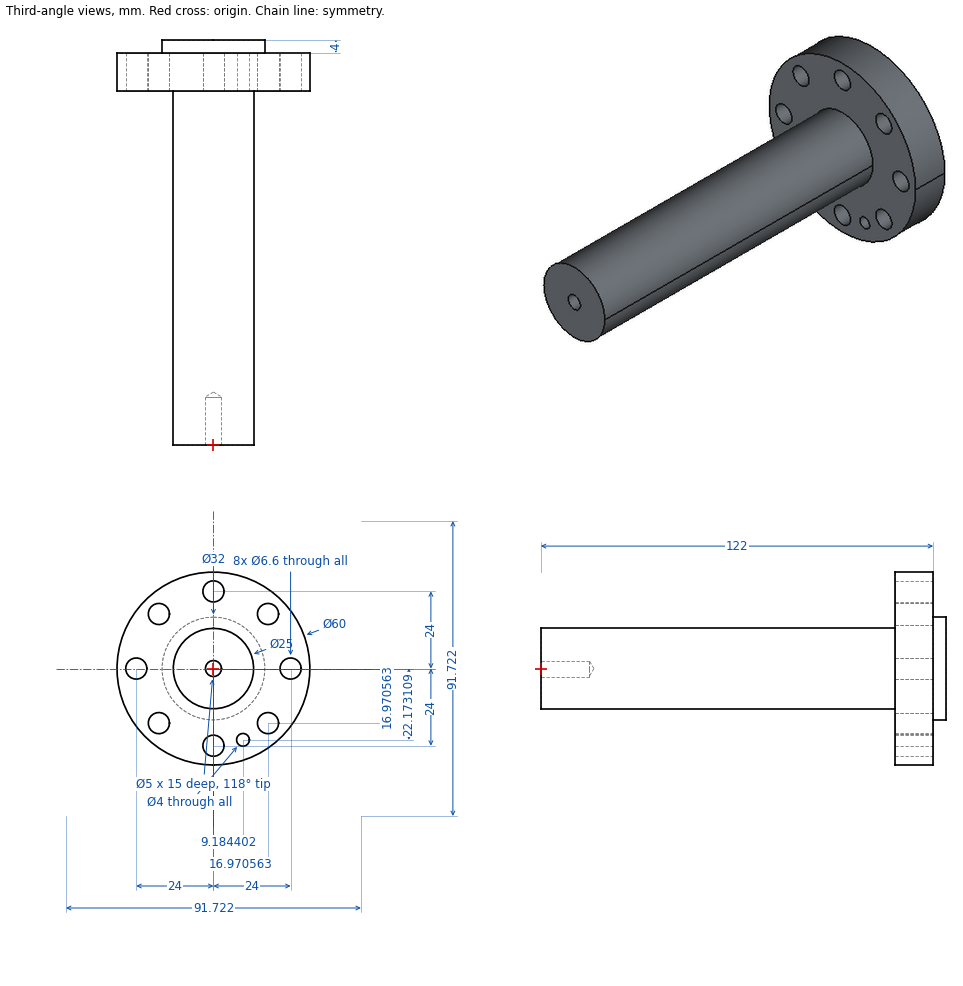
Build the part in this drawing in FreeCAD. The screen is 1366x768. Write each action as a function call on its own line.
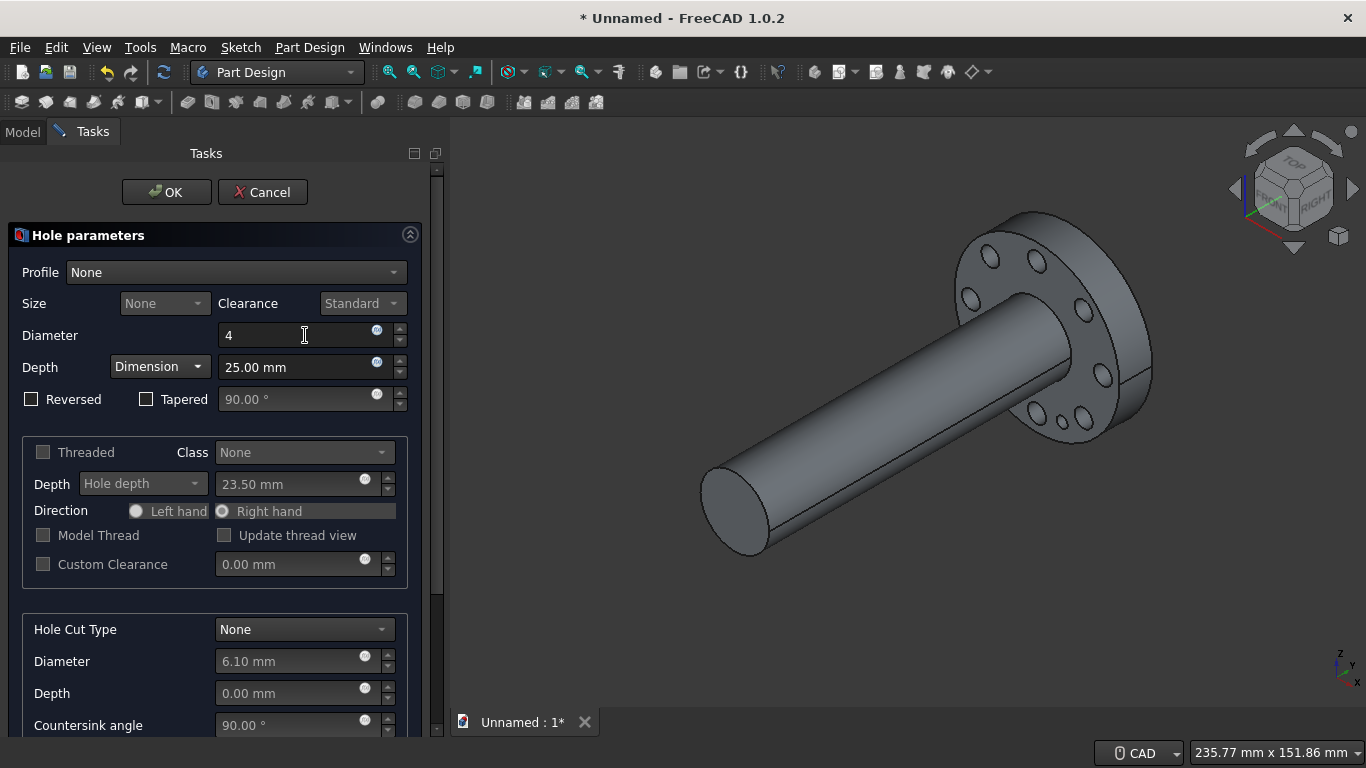
click(161, 366)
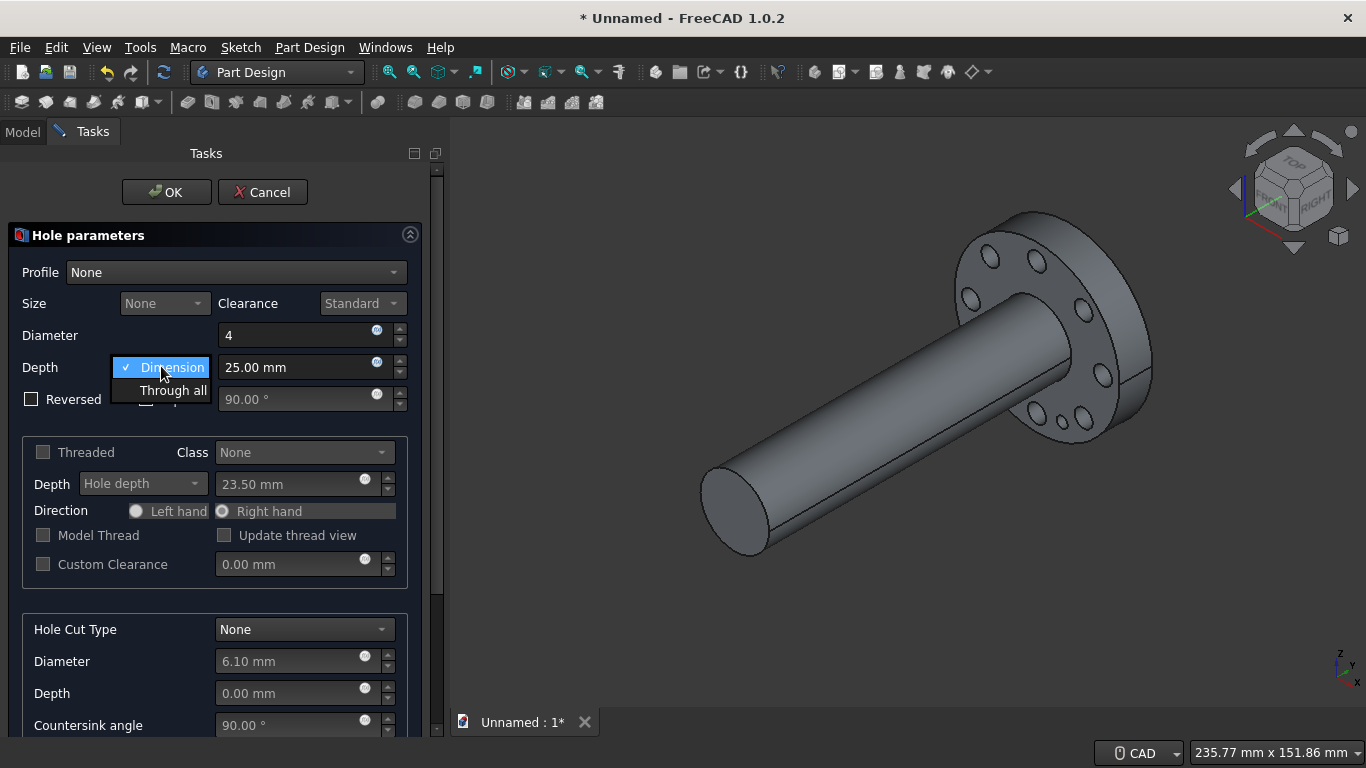
click(160, 390)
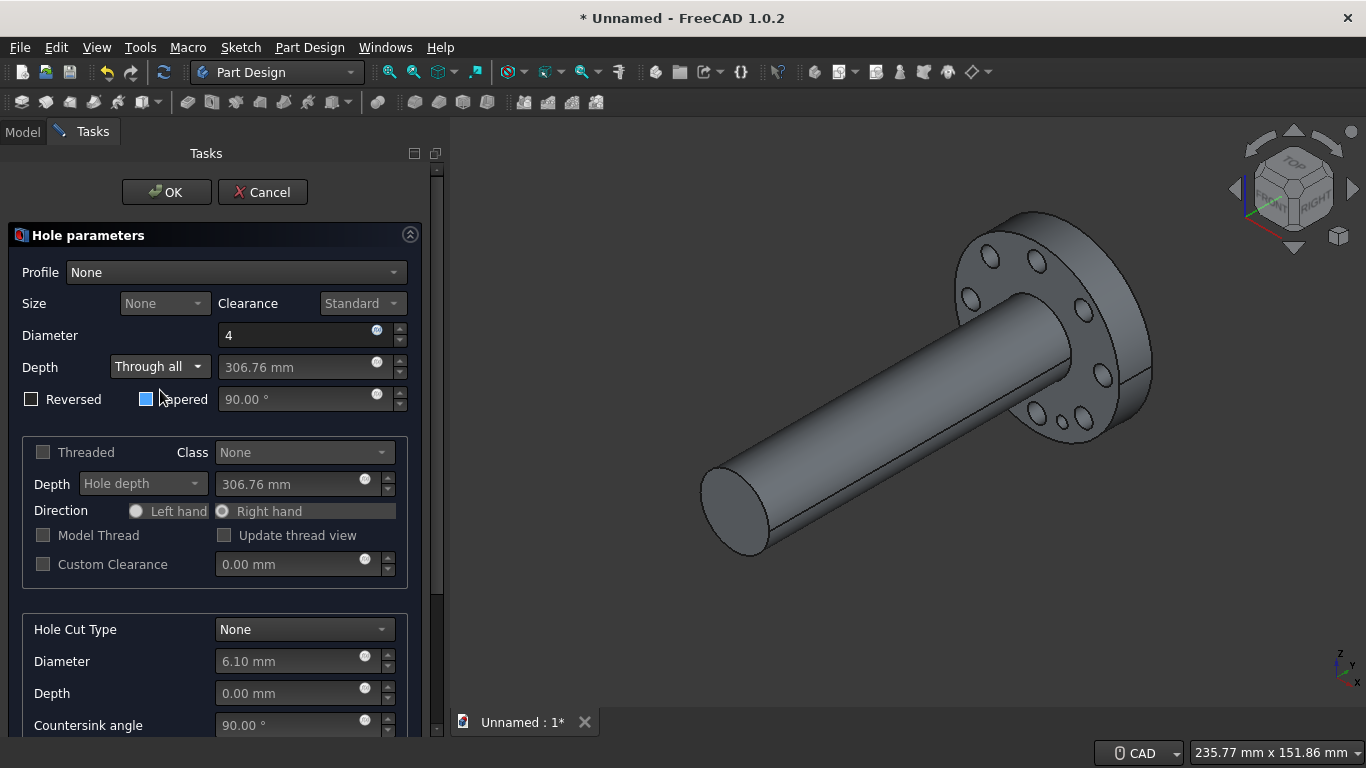
click(167, 192)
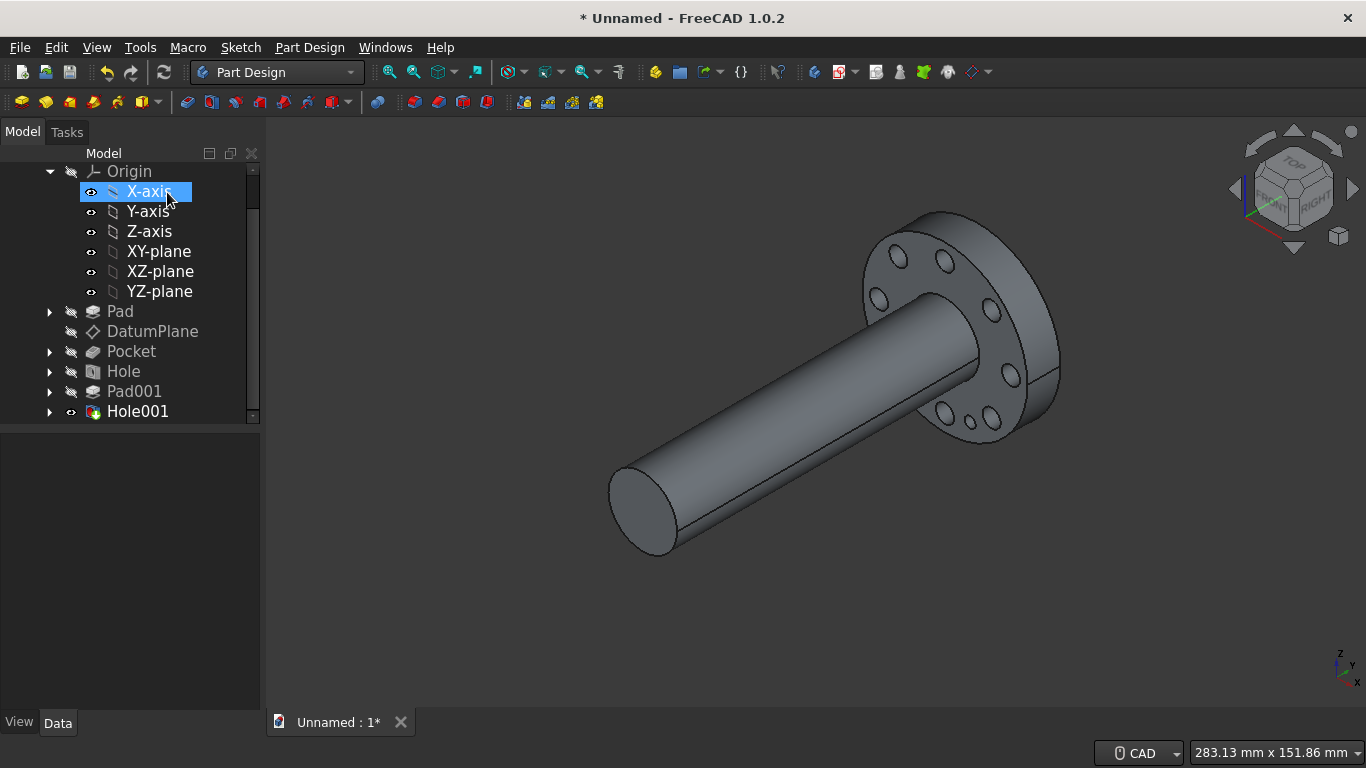
click(840, 72)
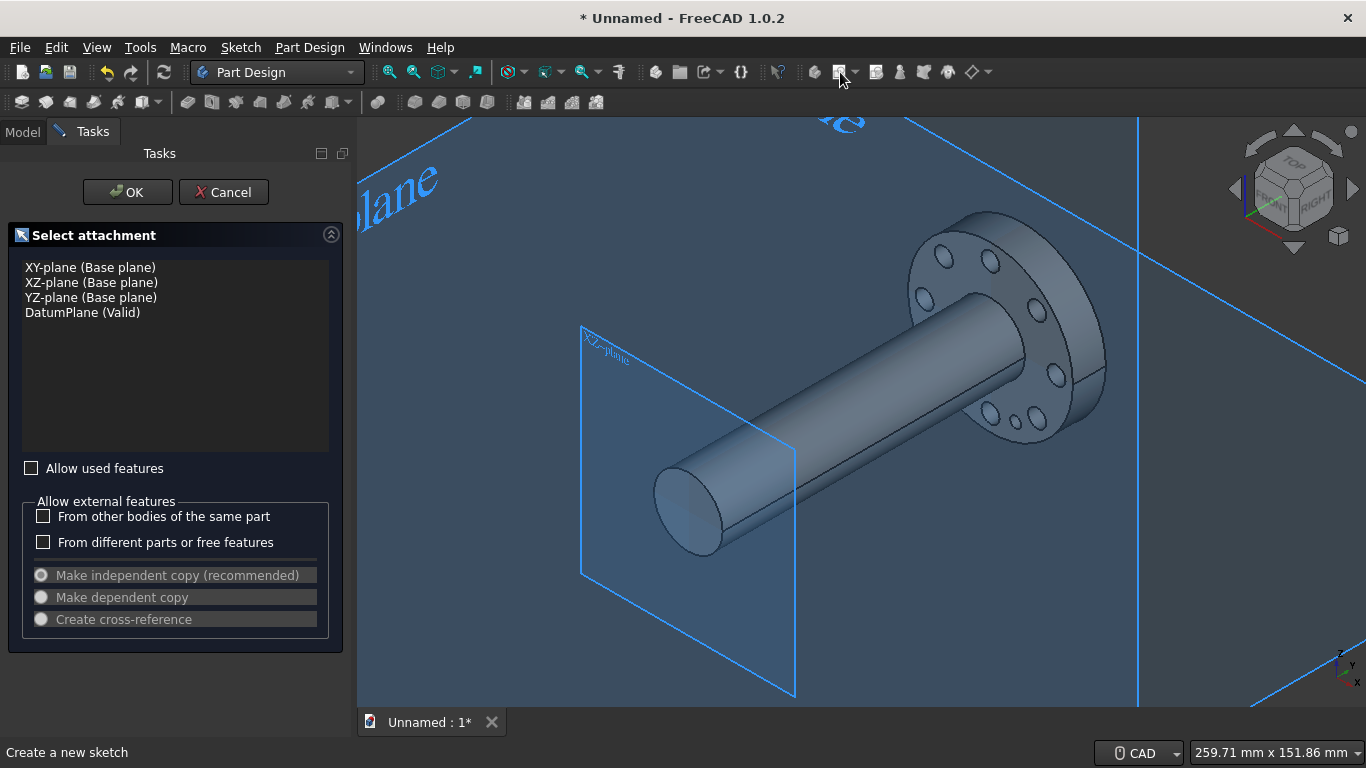
click(82, 282)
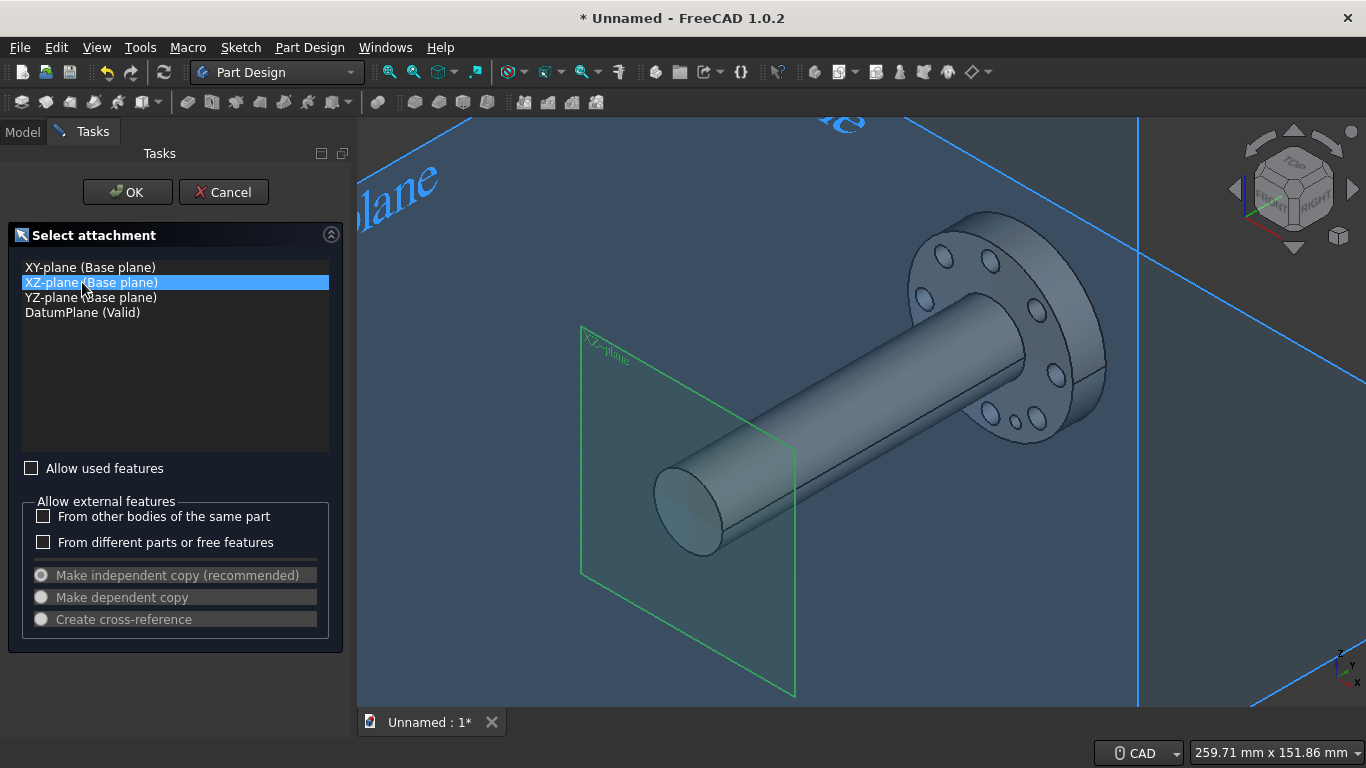
click(128, 192)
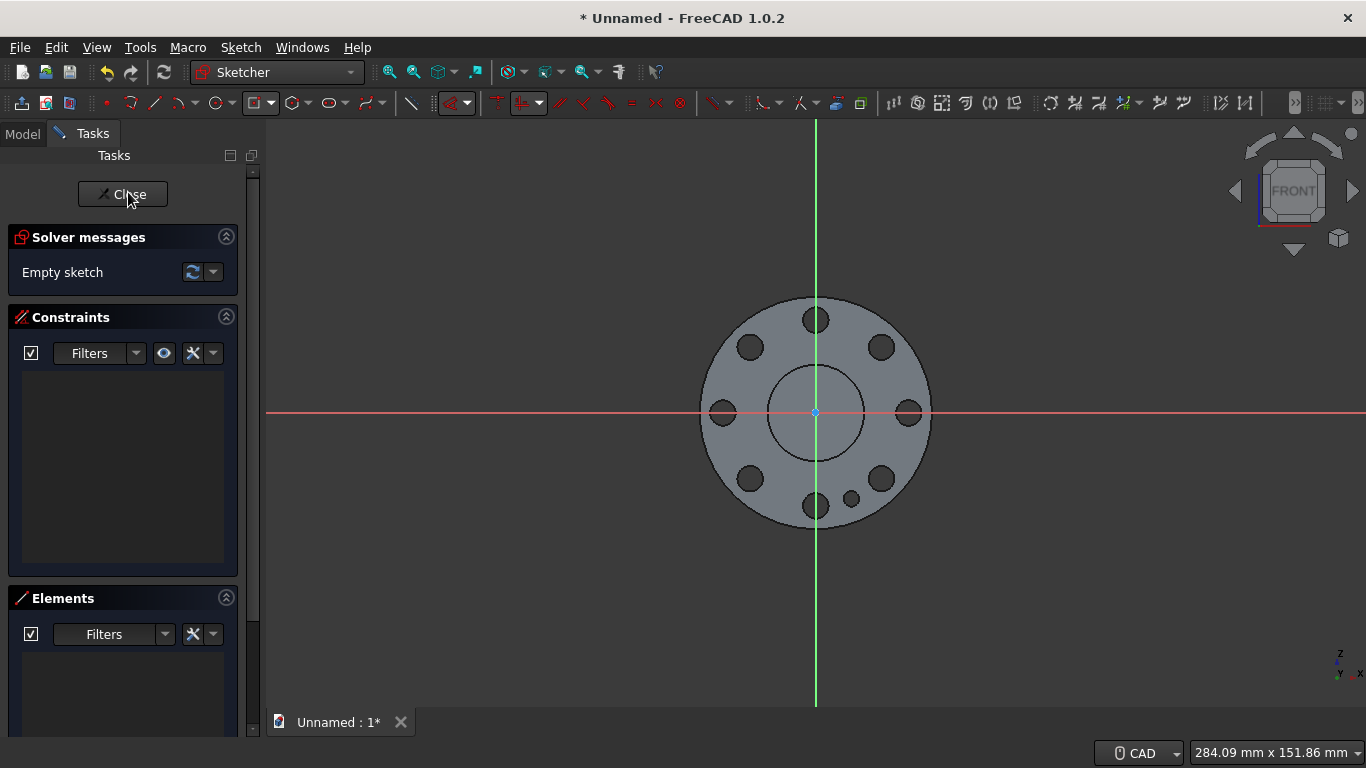
scroll(819, 413, up, 15)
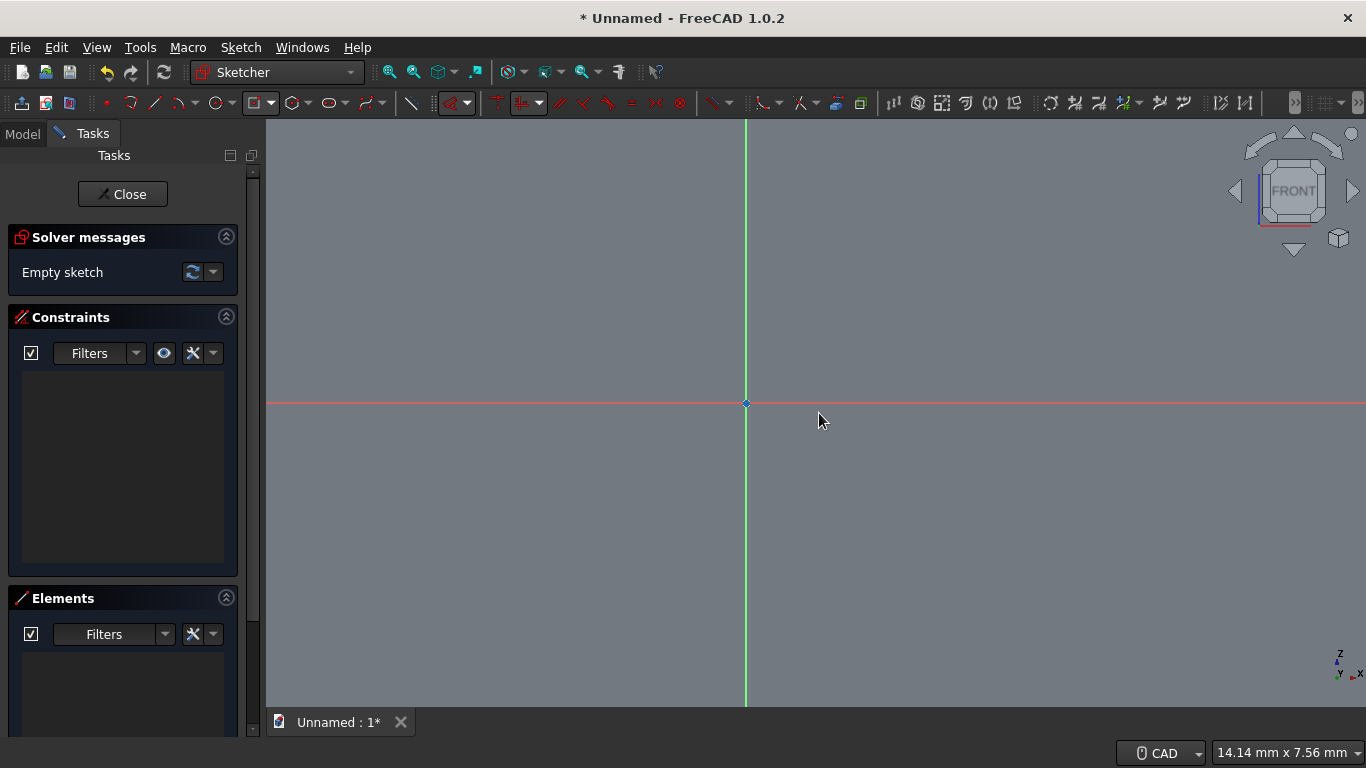
key(g)
key(c)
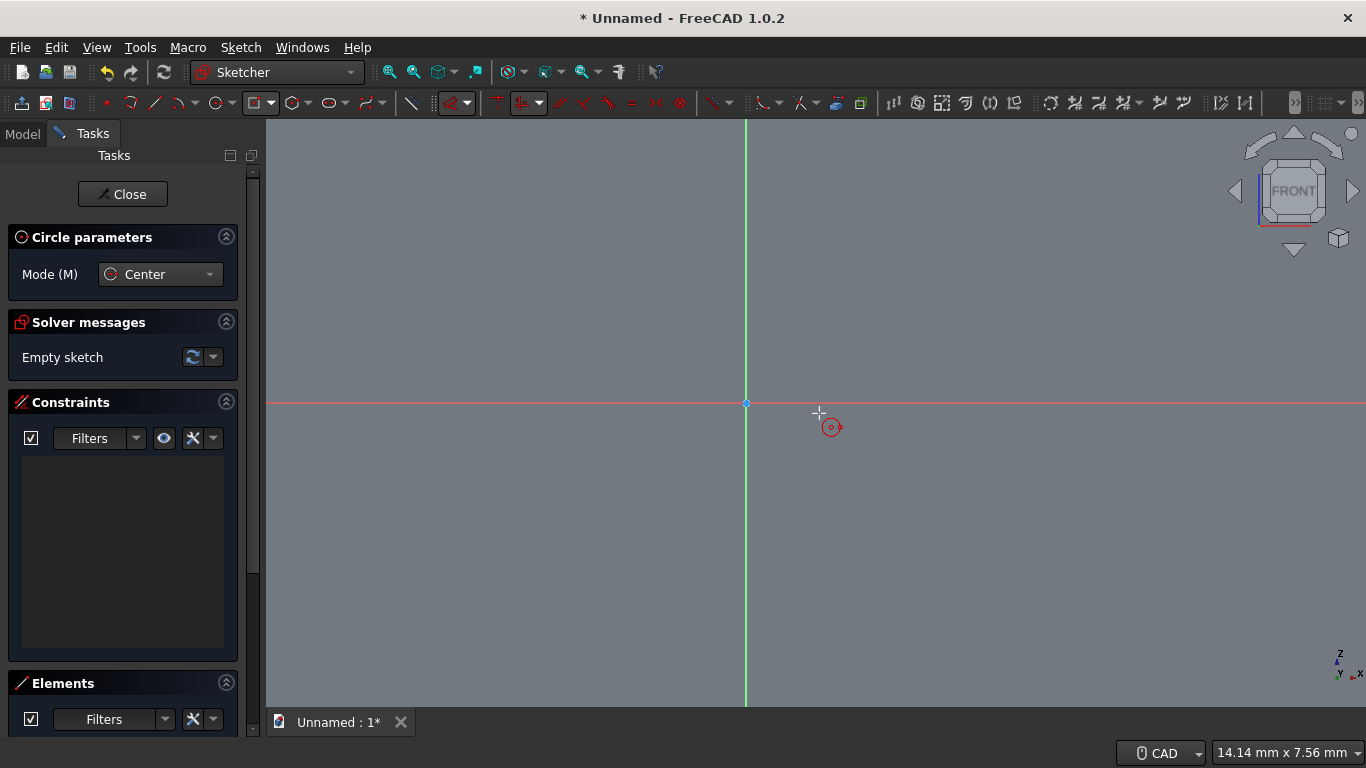
click(746, 403)
click(884, 266)
key(Escape)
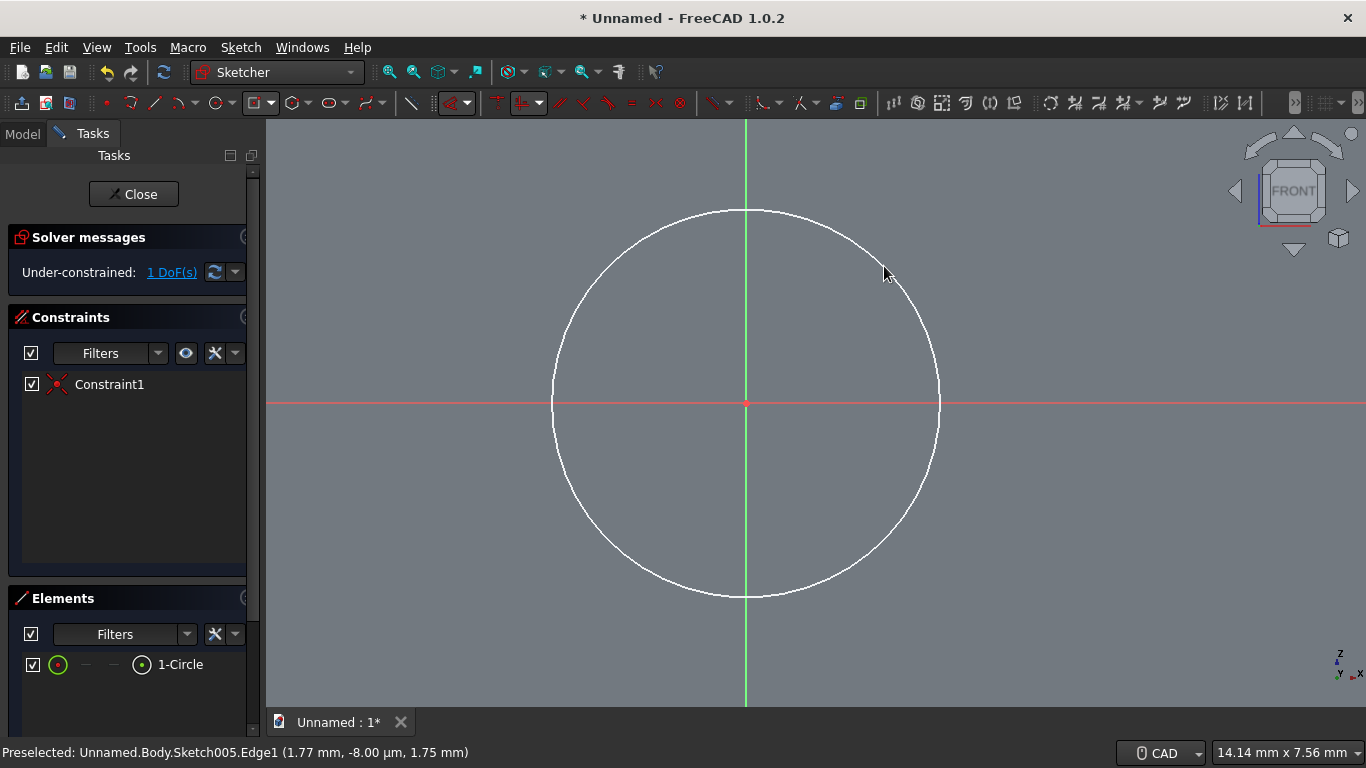
click(883, 266)